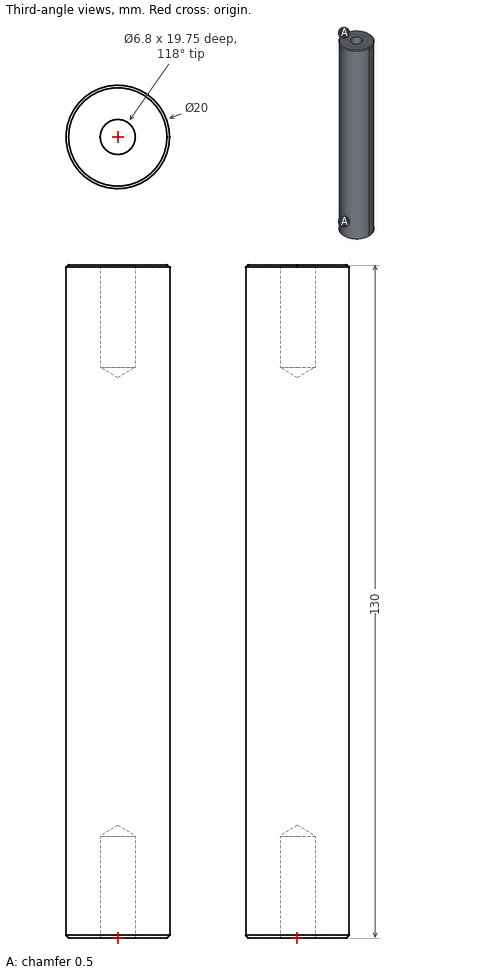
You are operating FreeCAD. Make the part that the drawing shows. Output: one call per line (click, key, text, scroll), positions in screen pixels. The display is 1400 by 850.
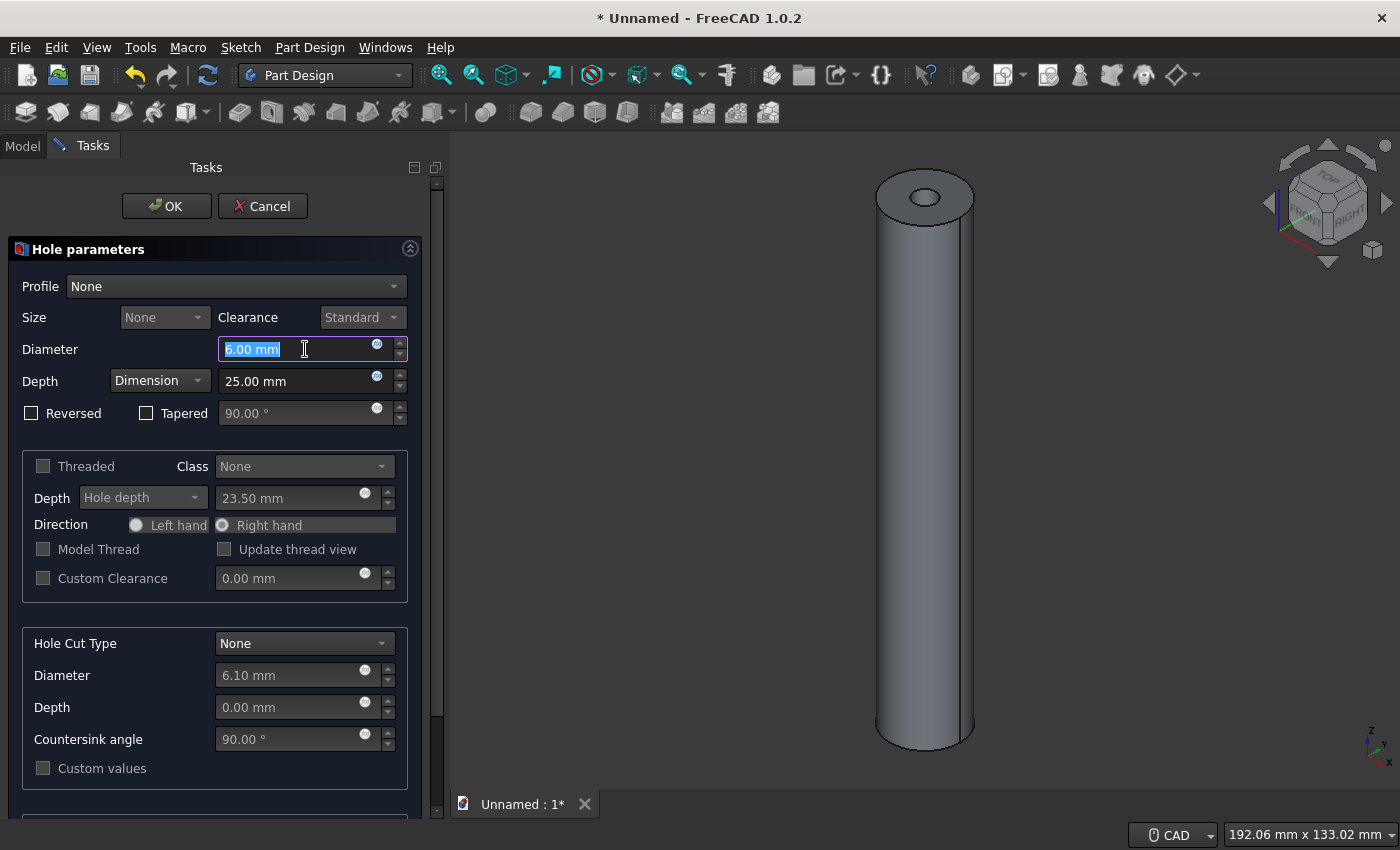
text(6.8)
key(Tab)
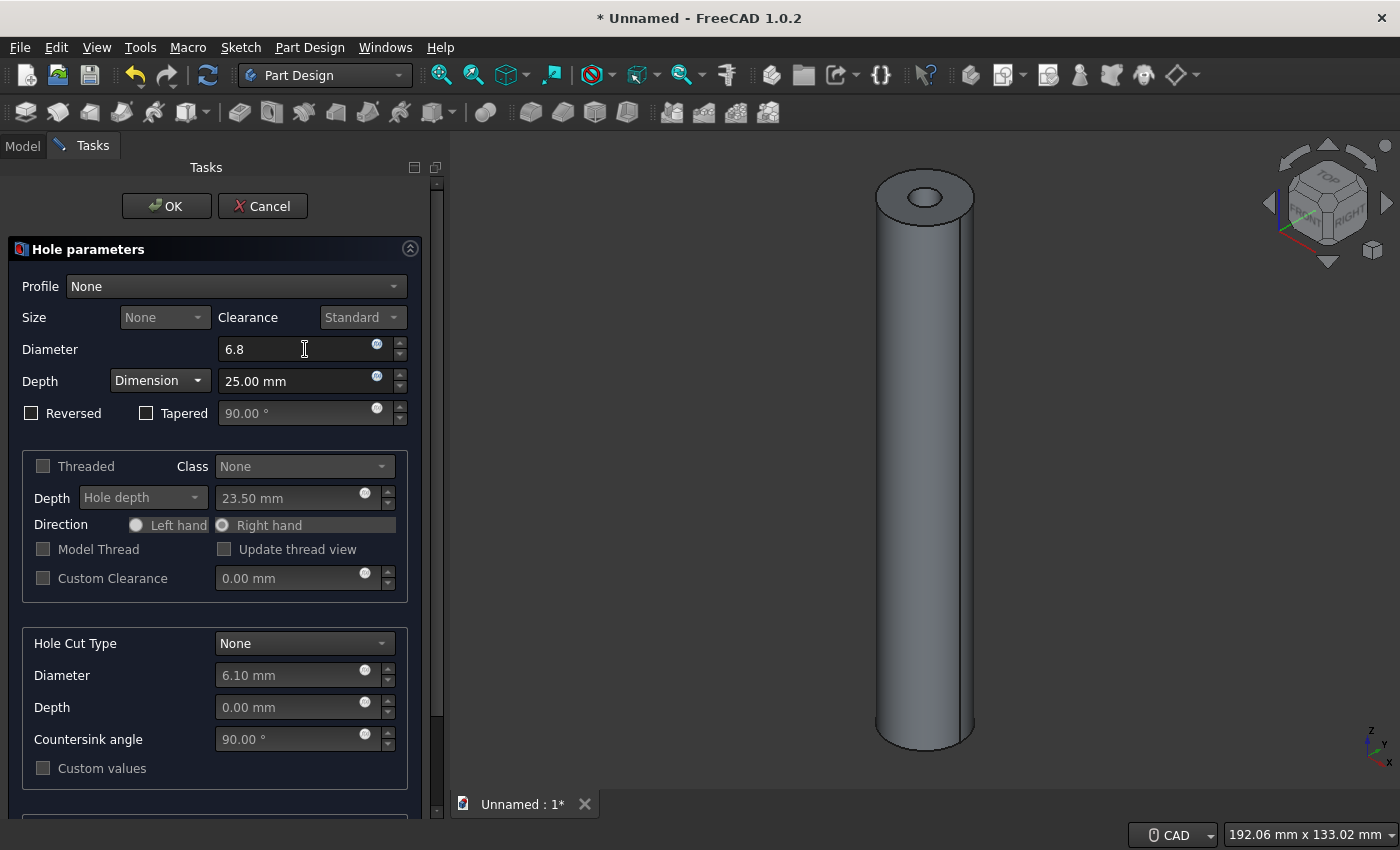
triple_click(305, 381)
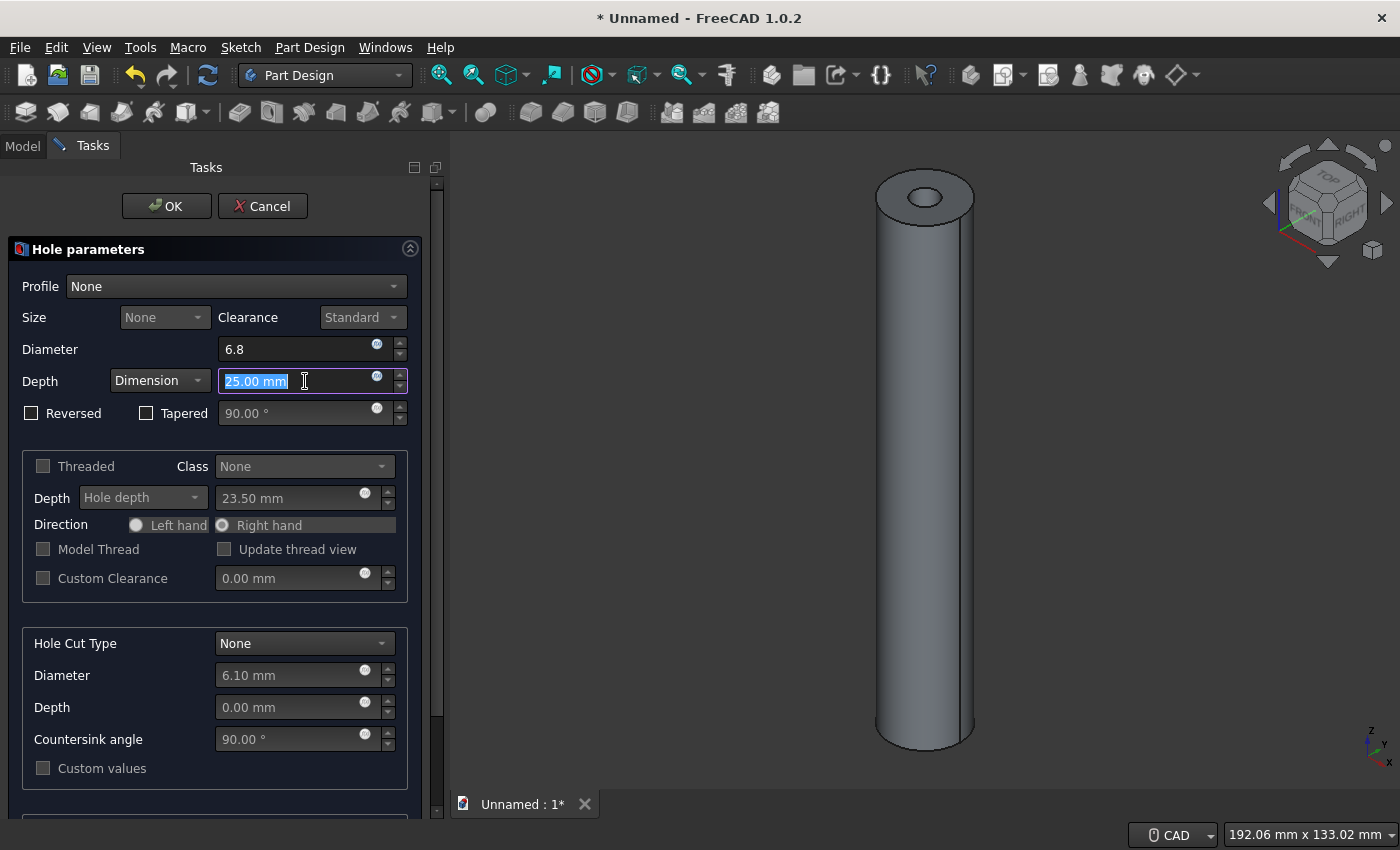
text(19.75)
key(Tab)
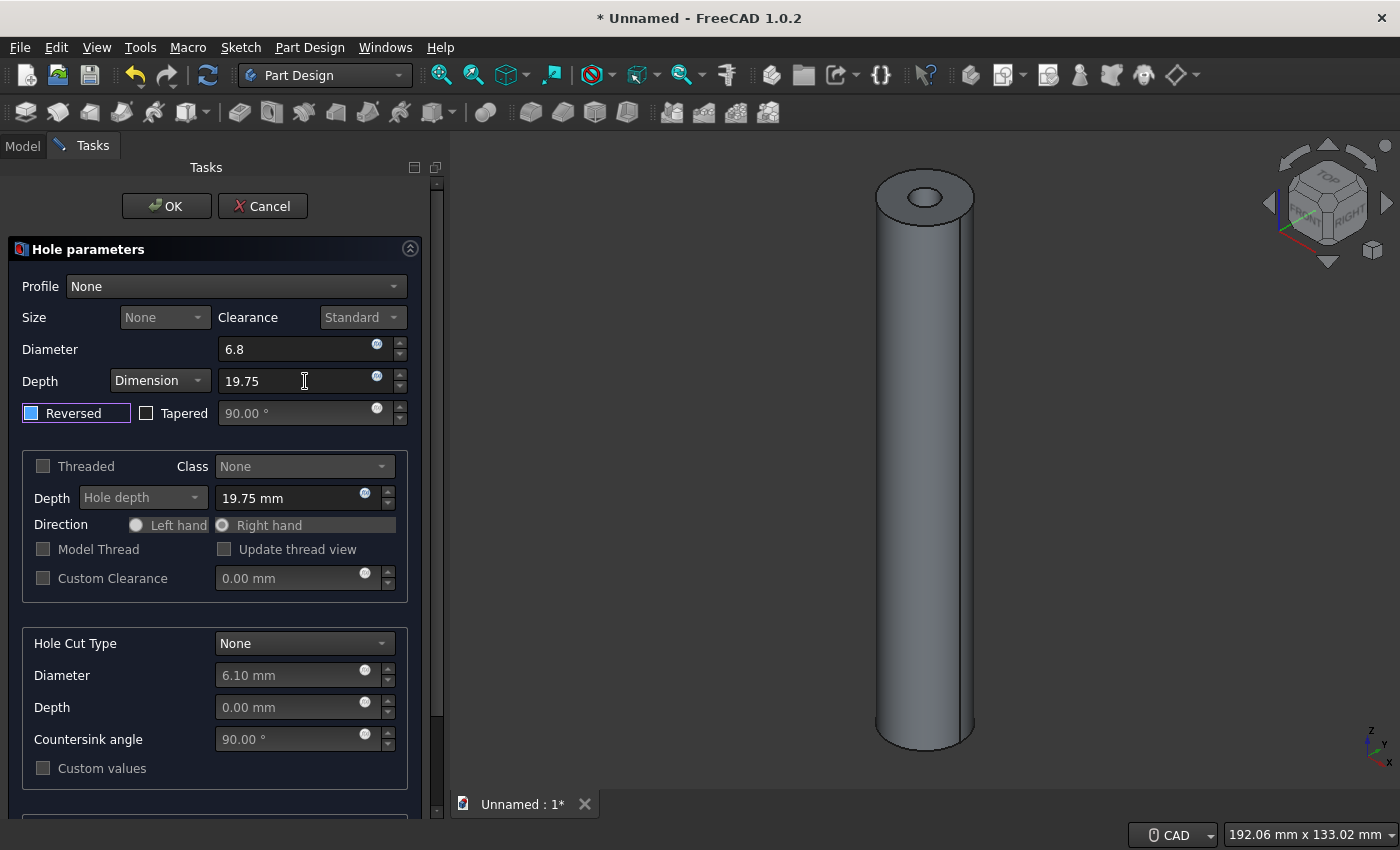
click(167, 206)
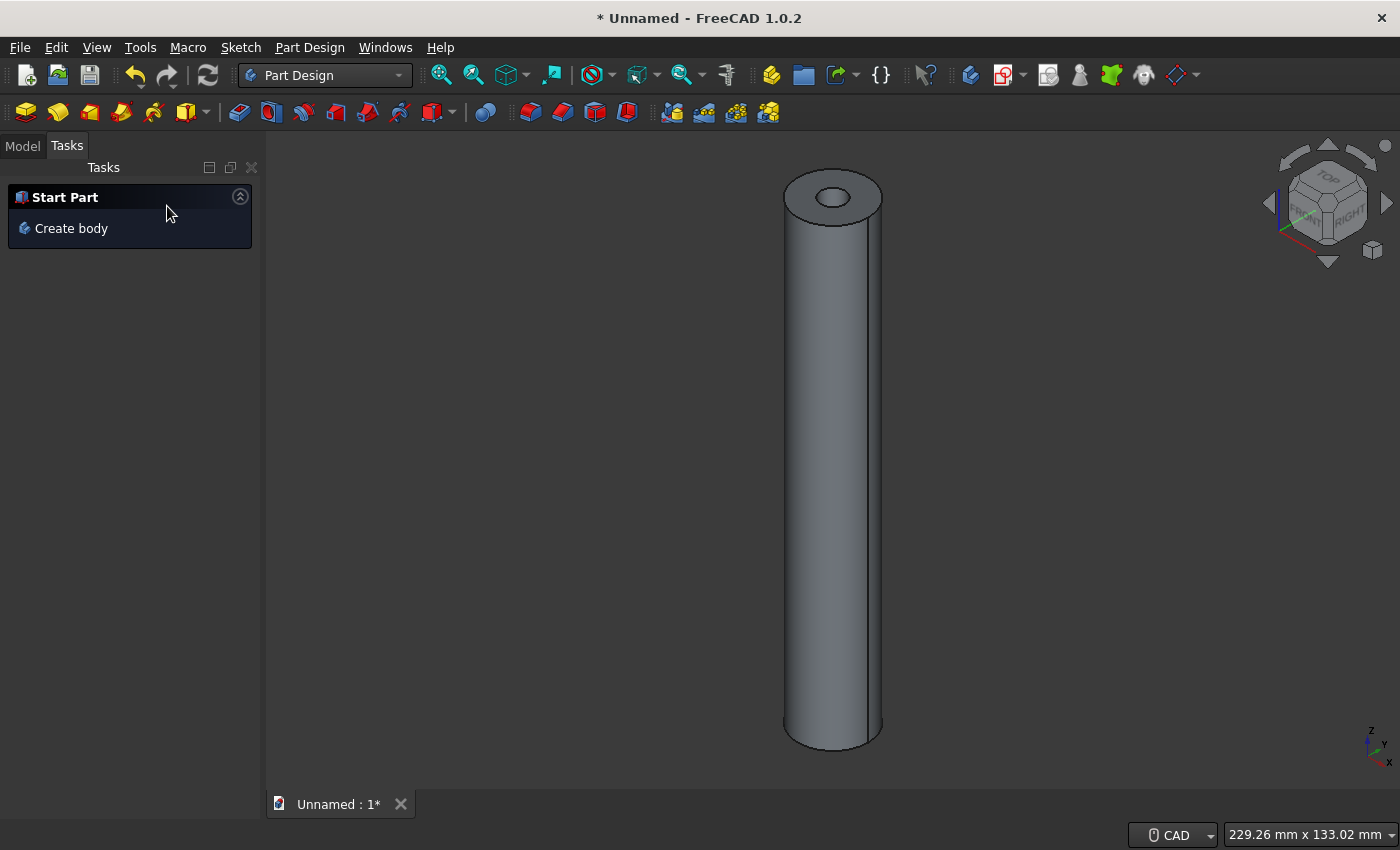
click(789, 209)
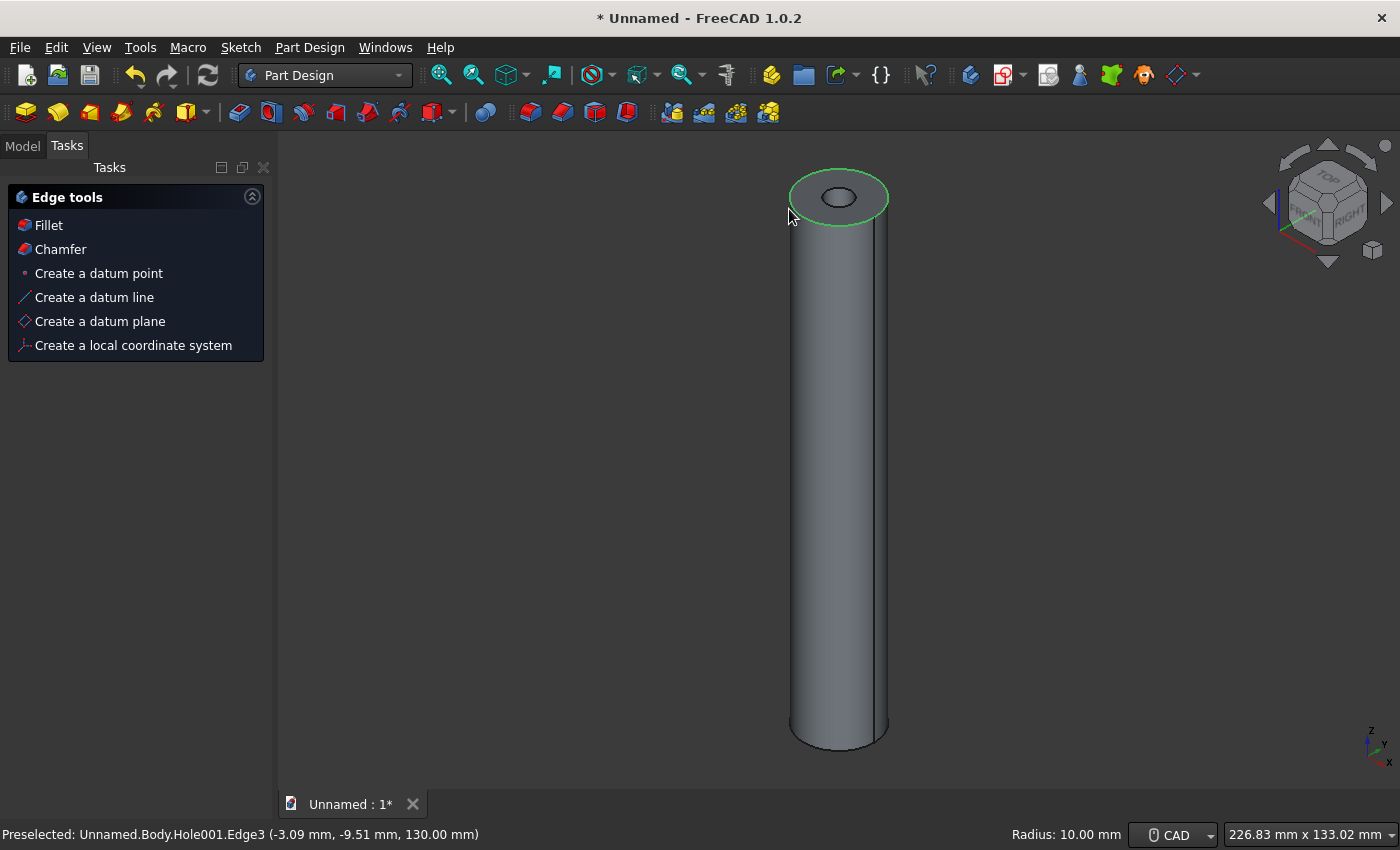
key(2)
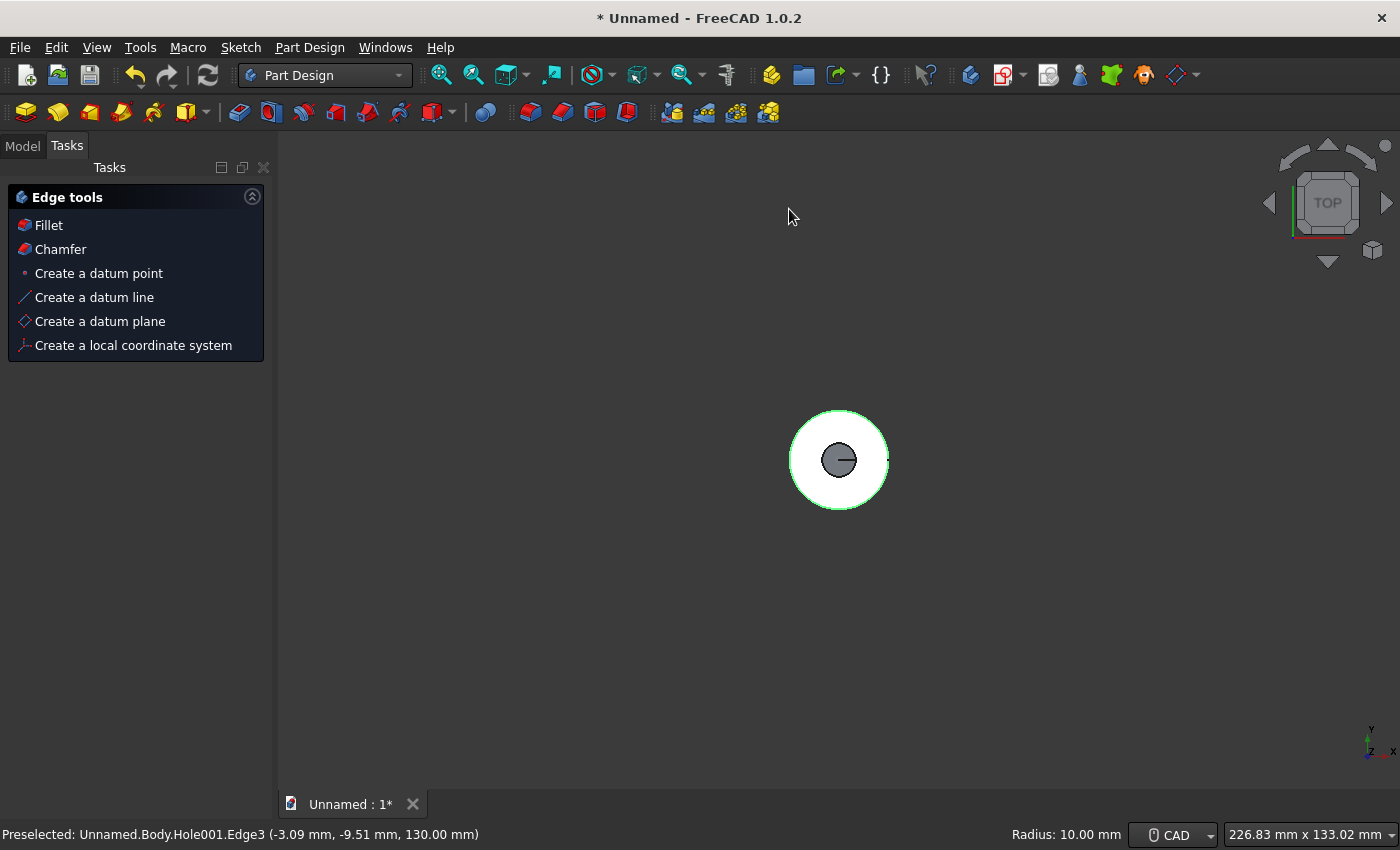
click(442, 76)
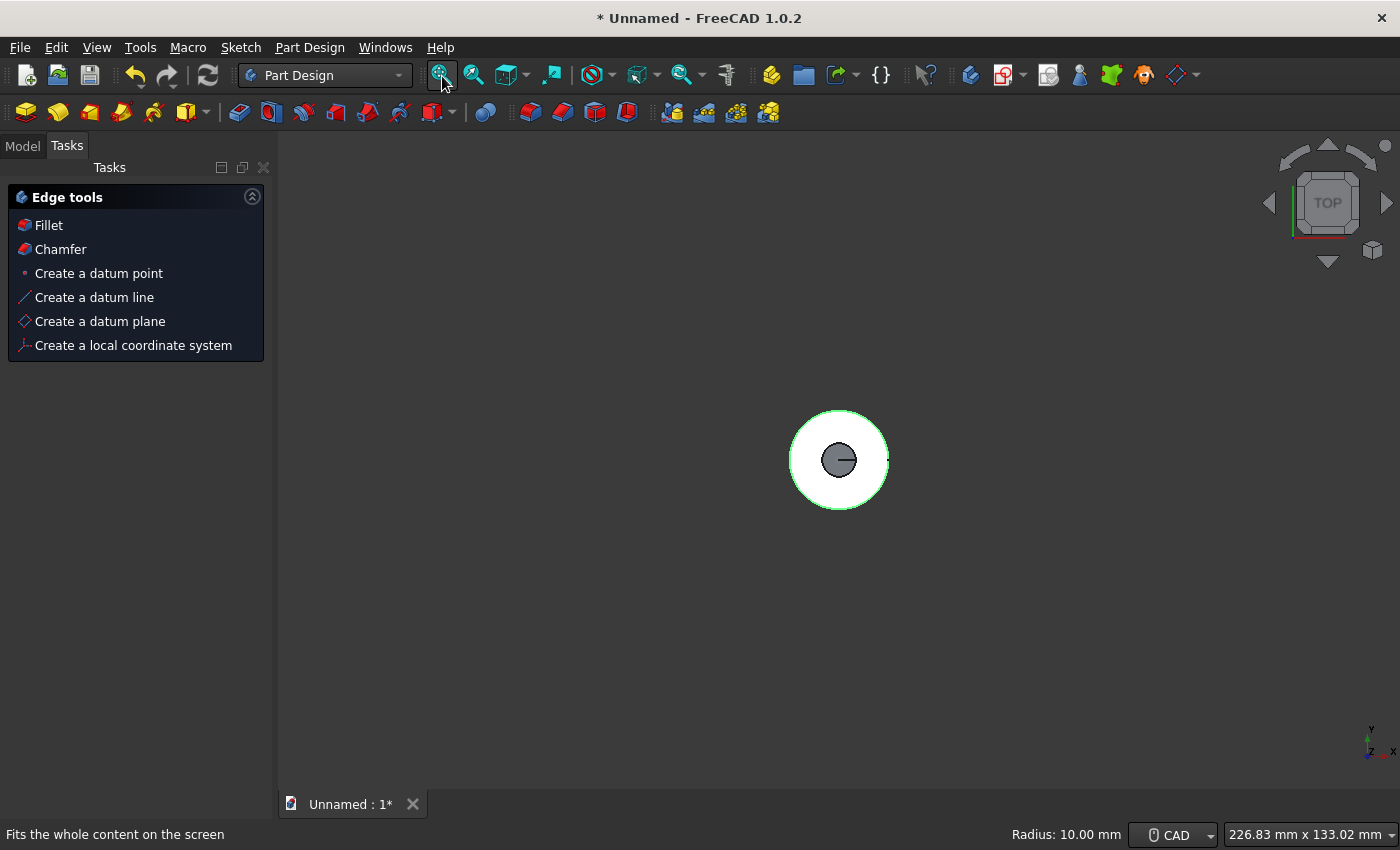
key(0)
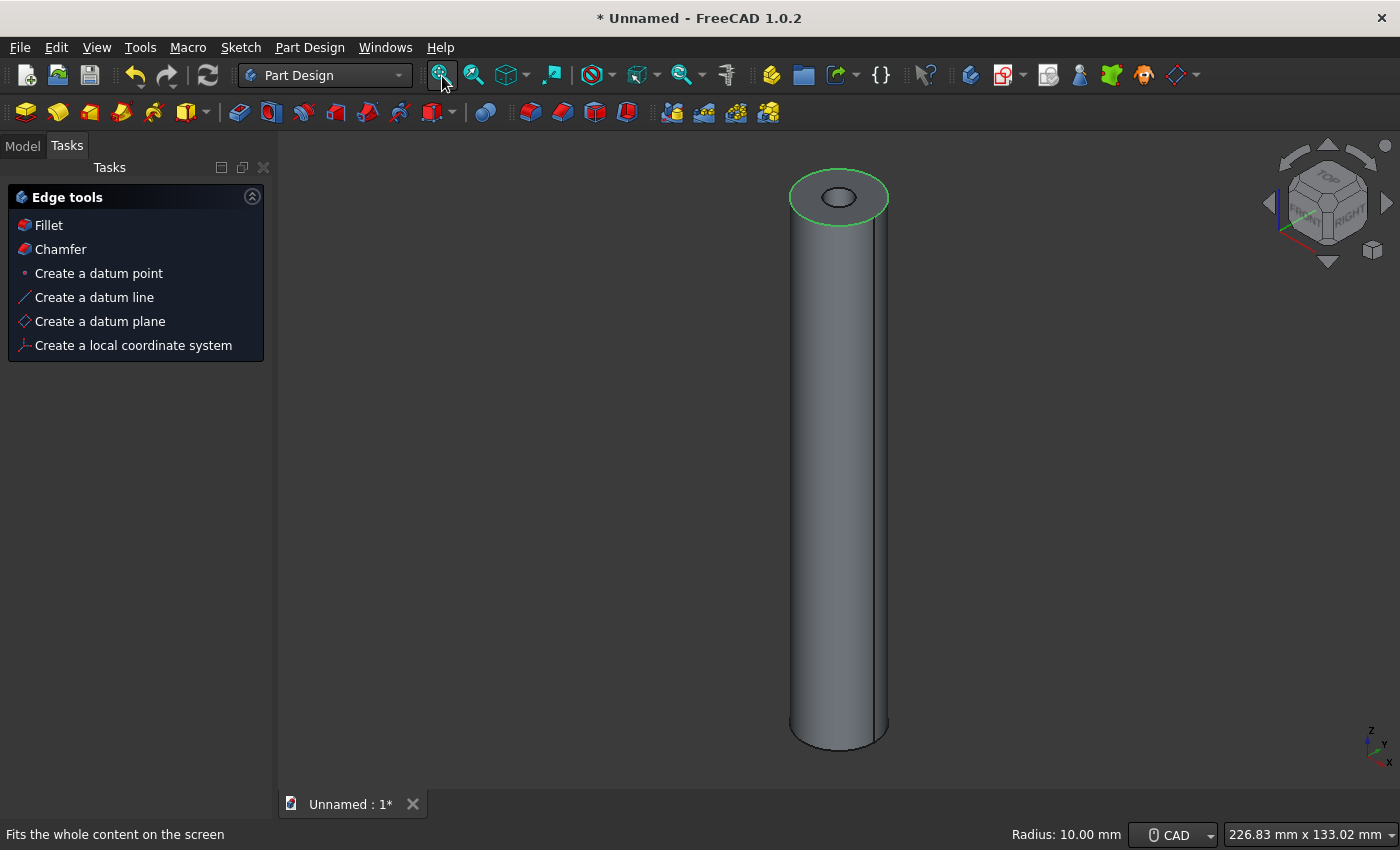
key(1)